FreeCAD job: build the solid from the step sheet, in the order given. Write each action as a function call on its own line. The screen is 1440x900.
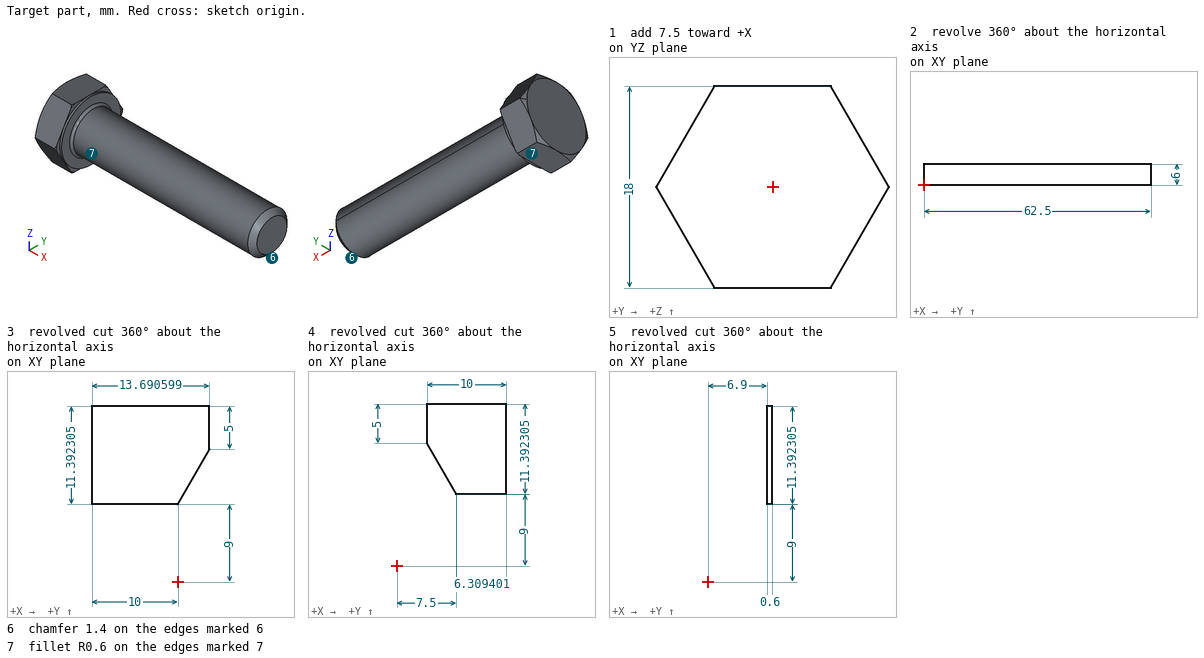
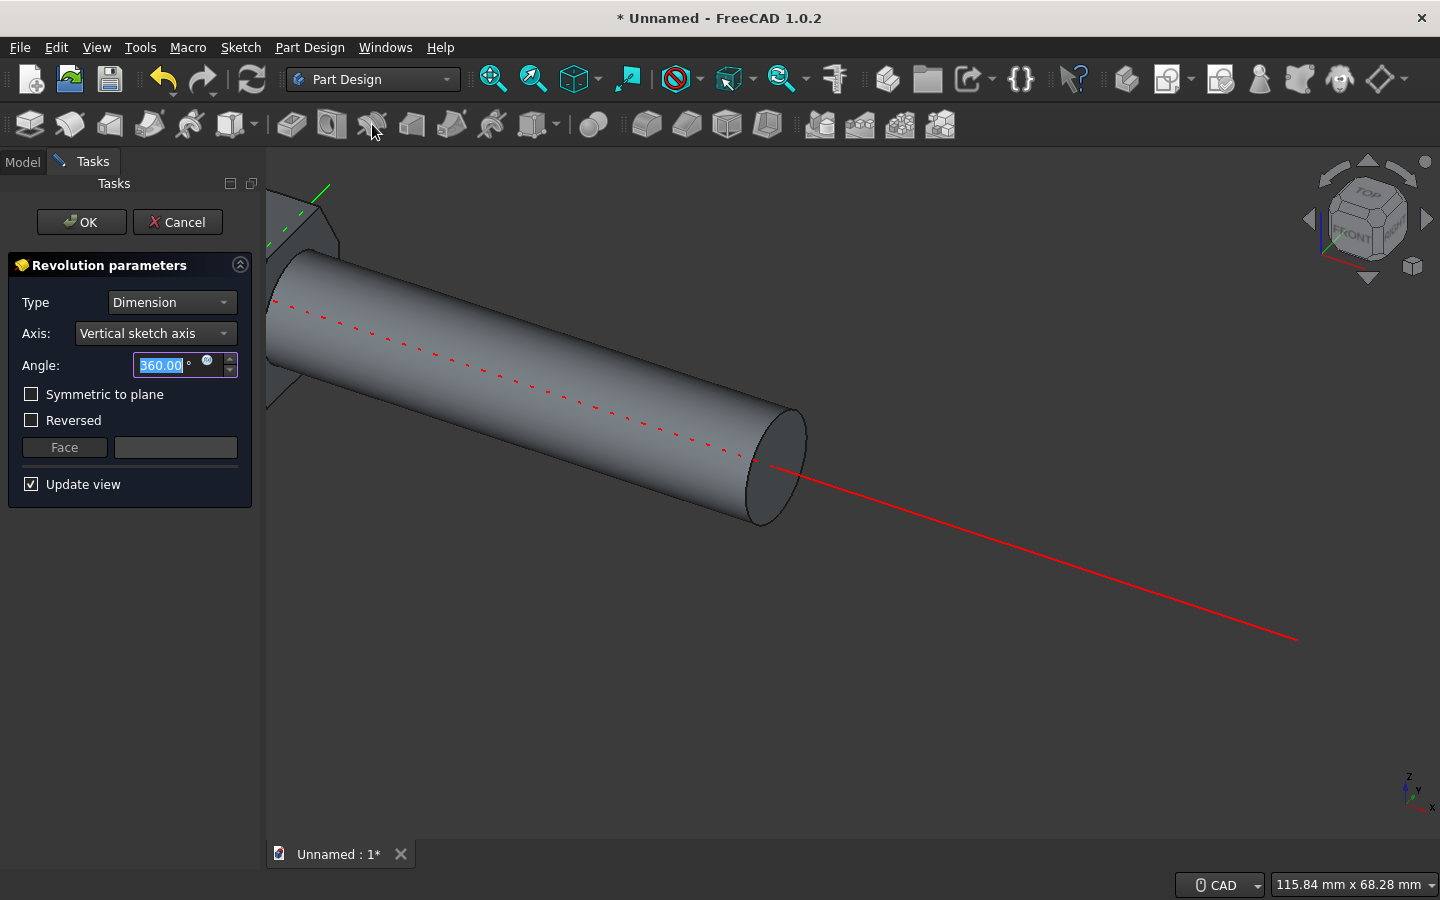
click(156, 334)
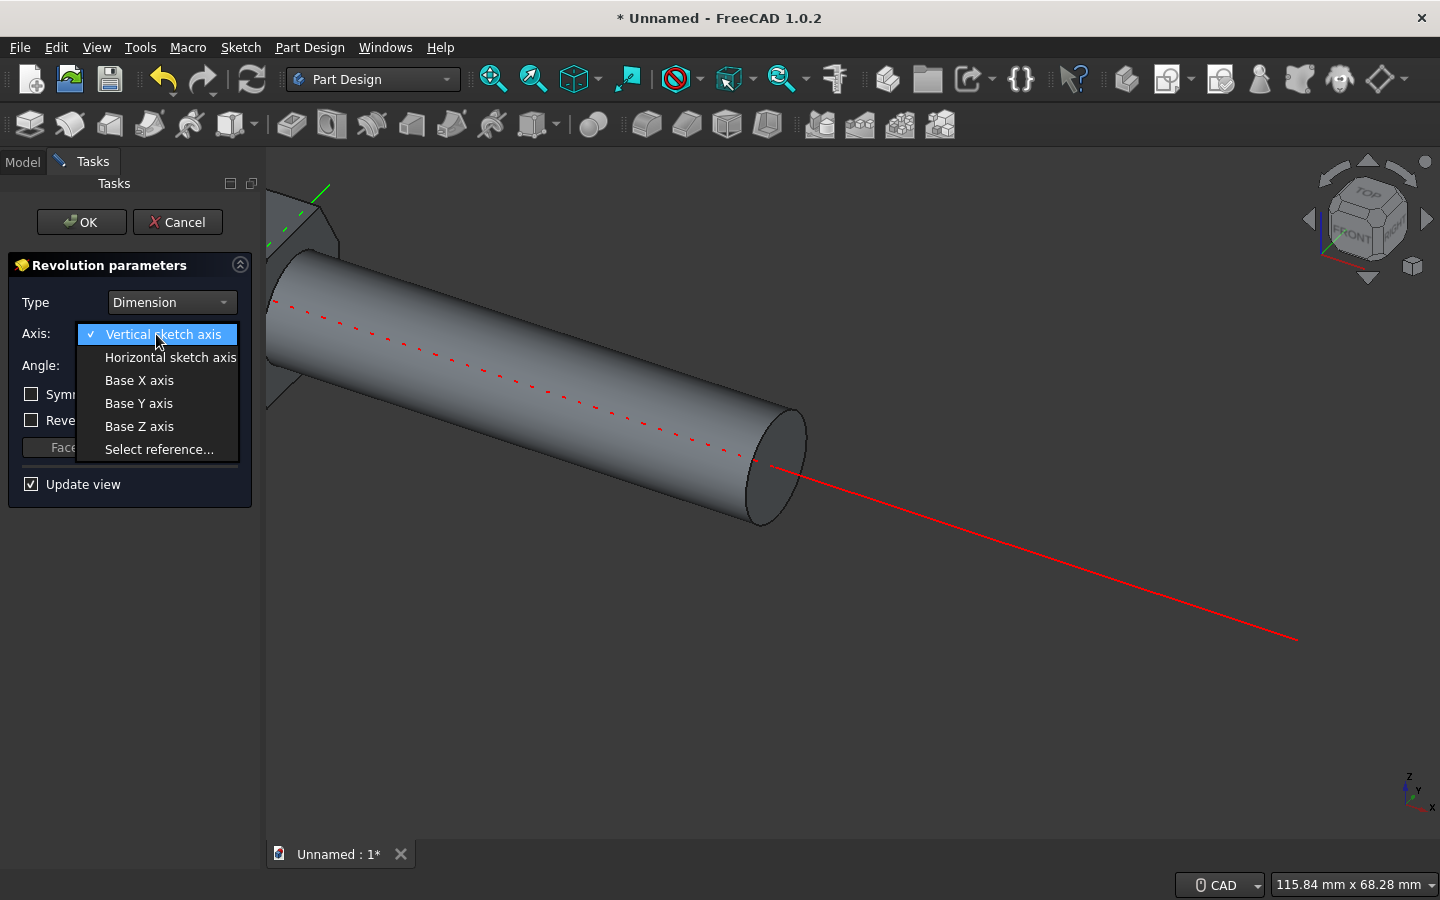
click(156, 358)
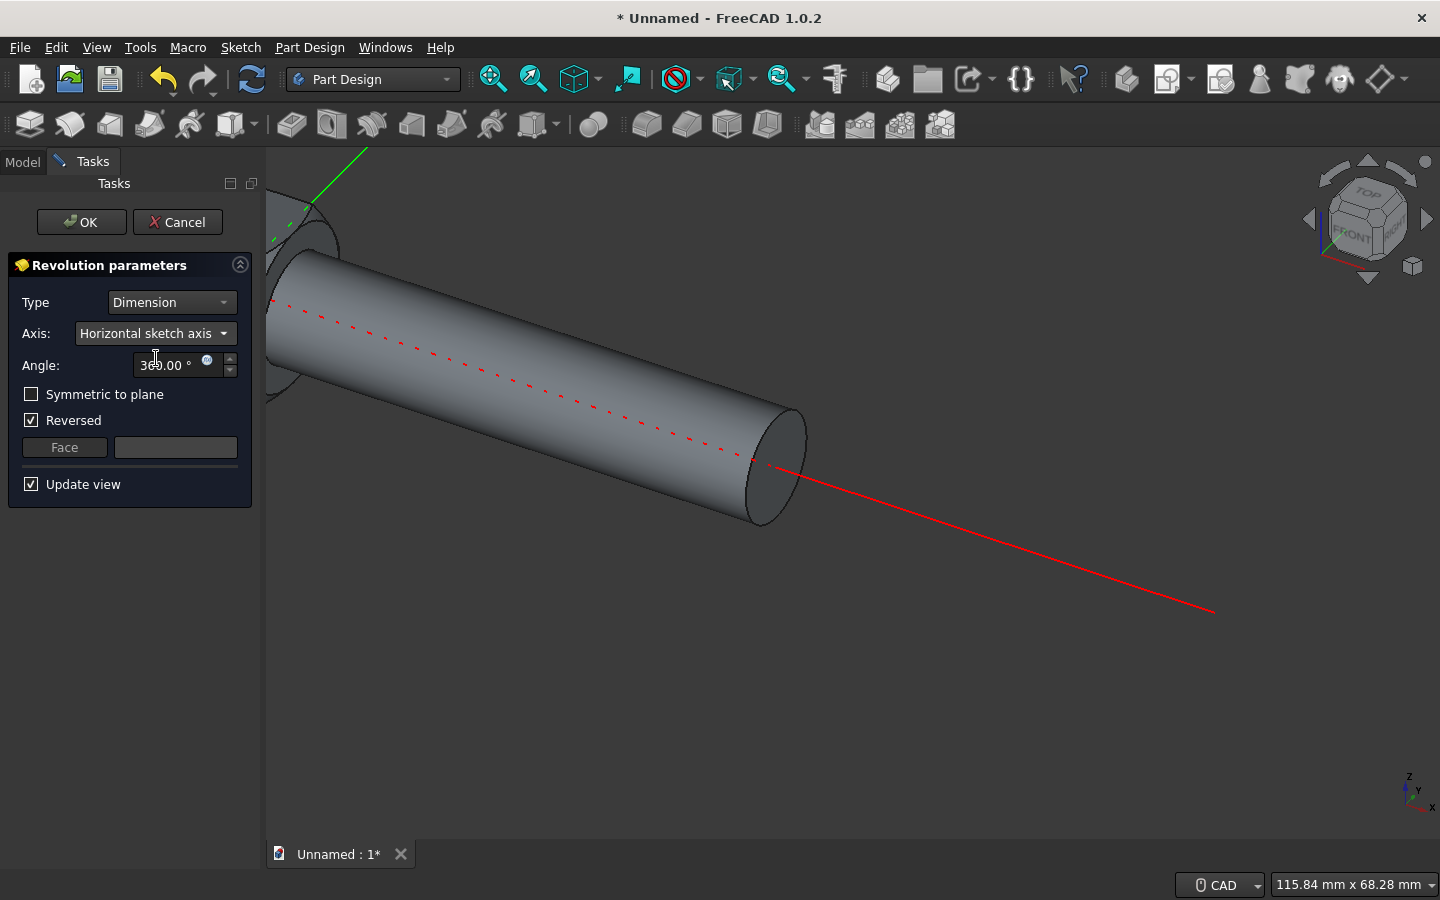
click(82, 222)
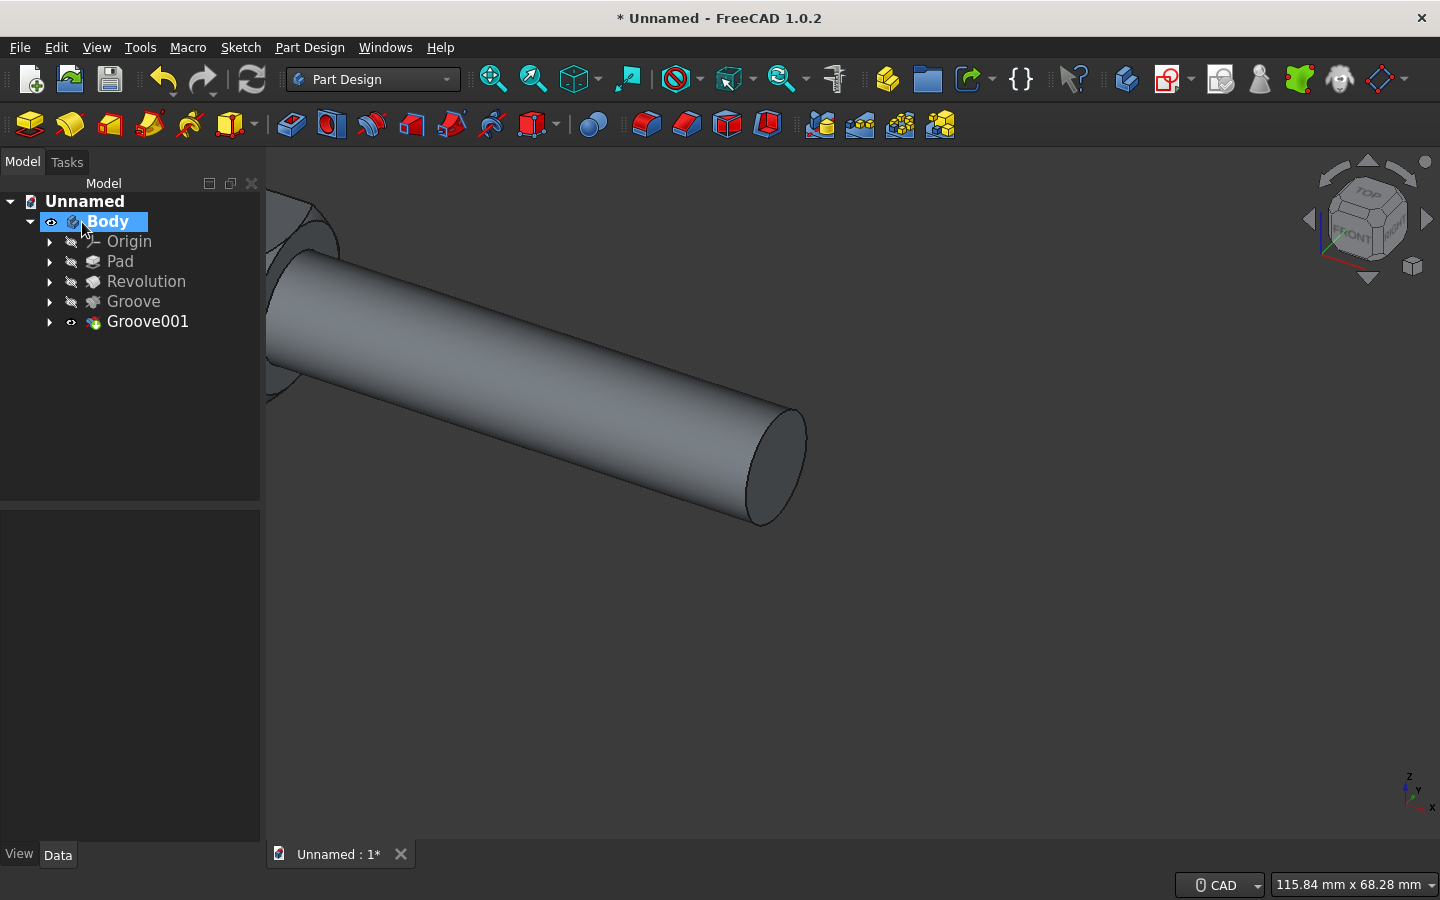
click(494, 80)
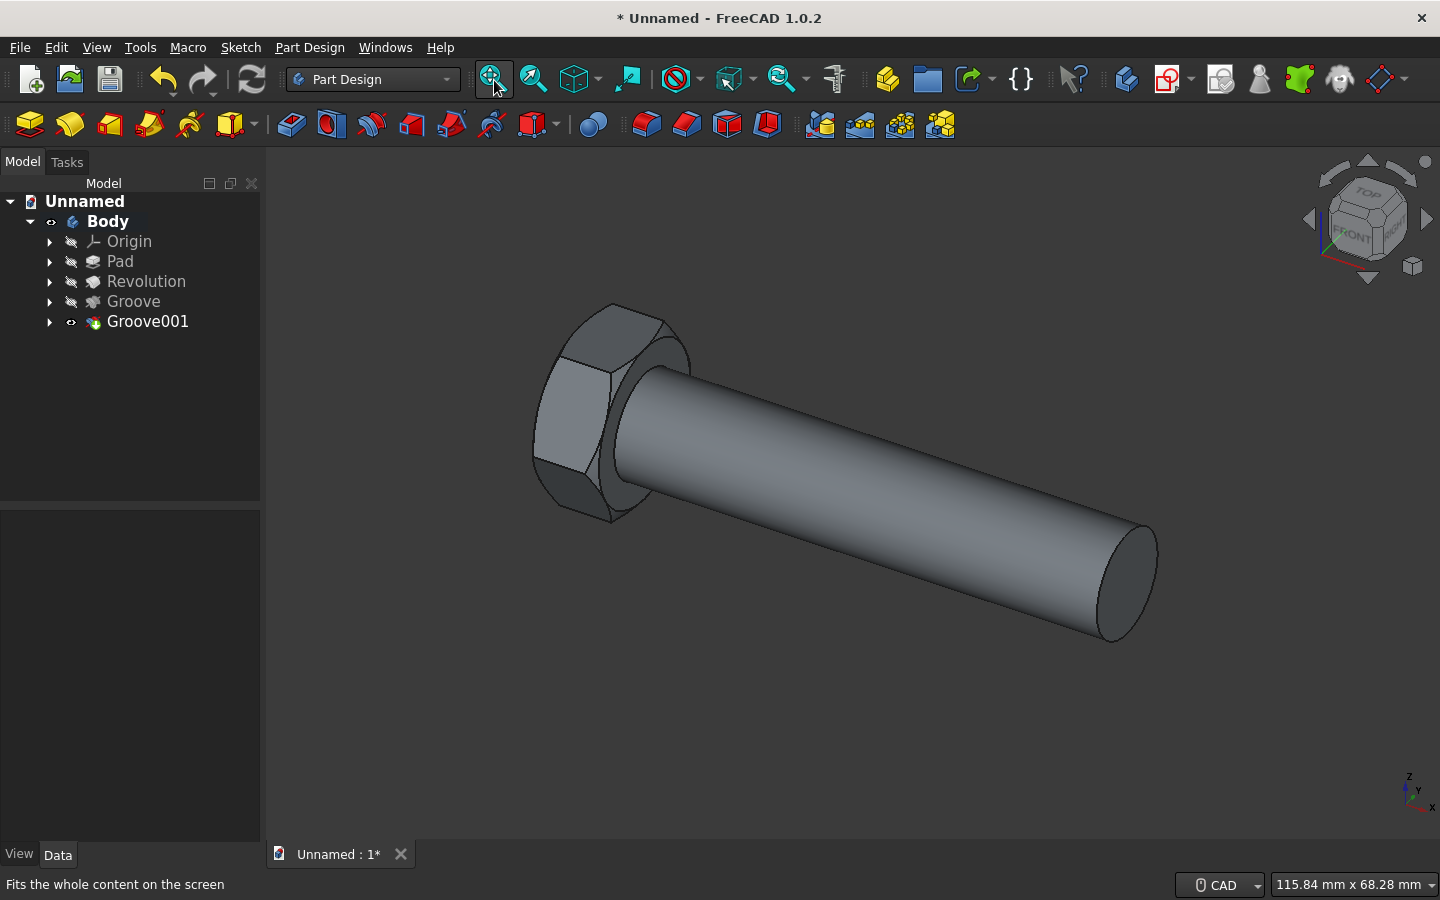
click(1168, 80)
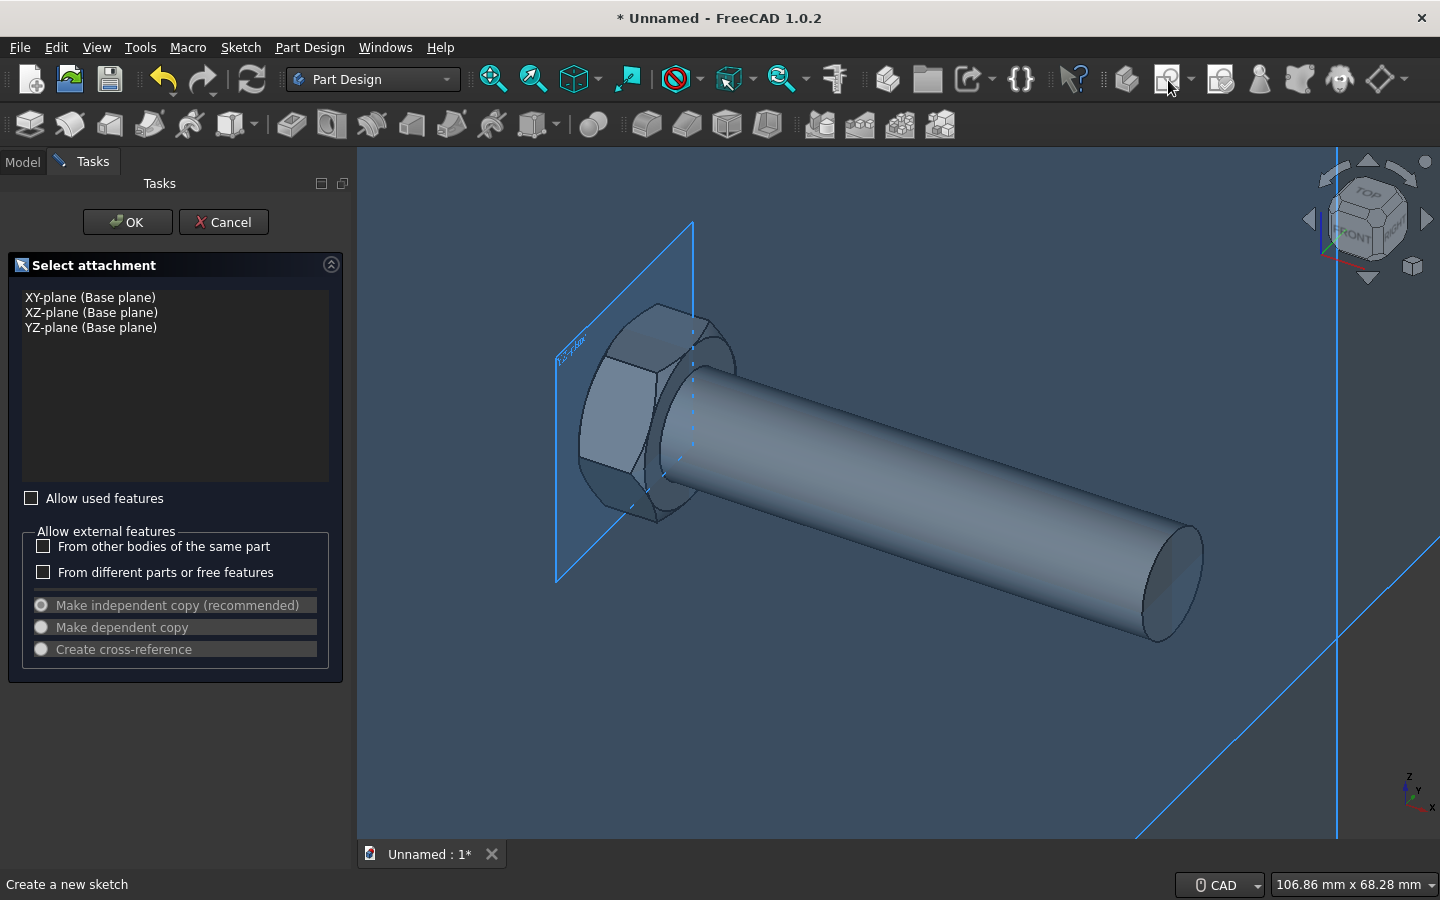
click(82, 298)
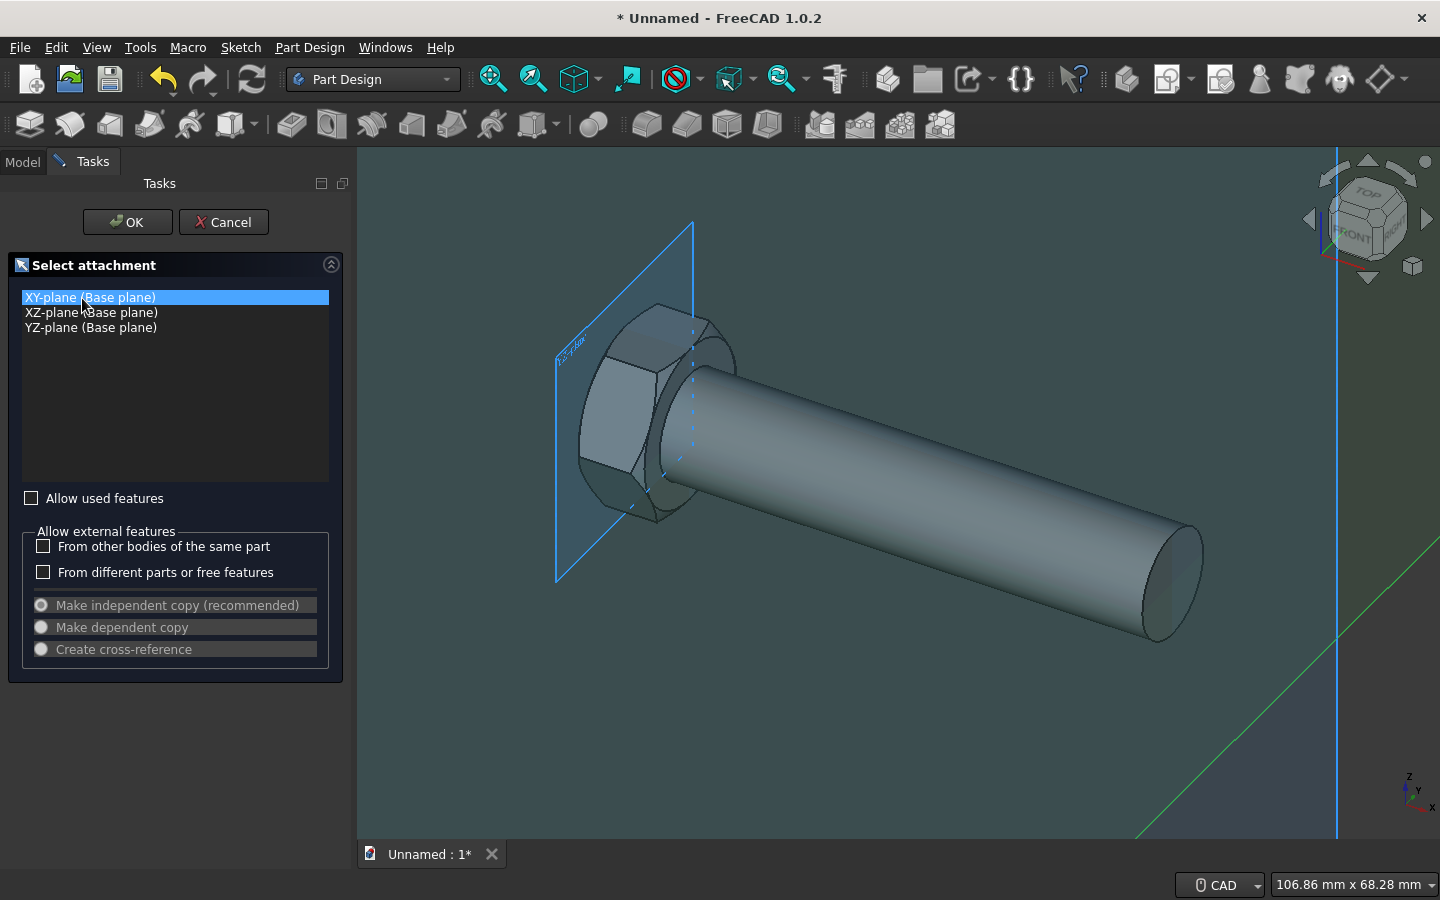
click(128, 222)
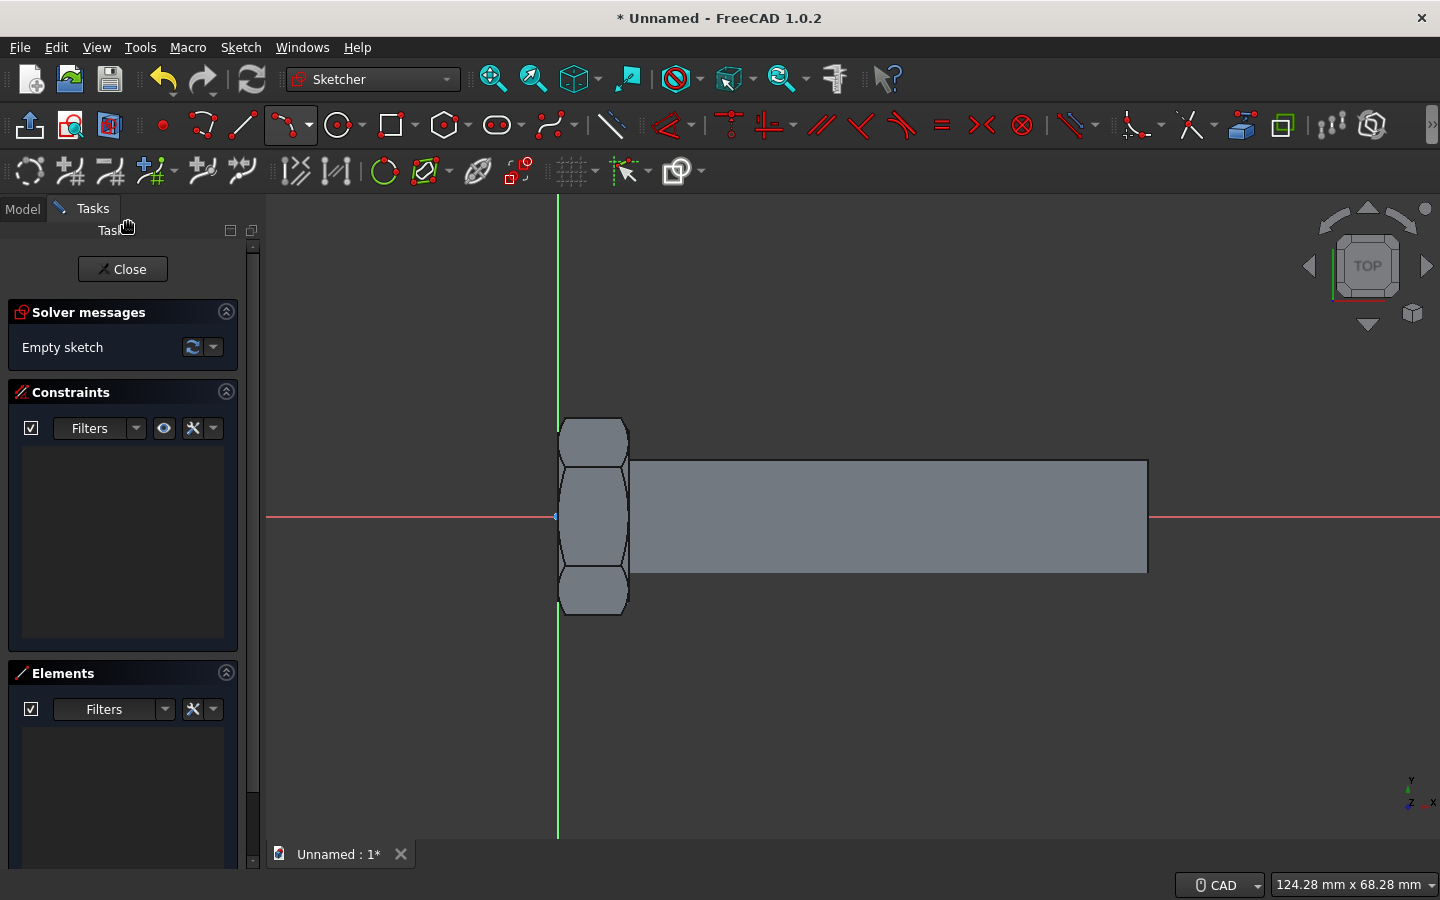
click(110, 126)